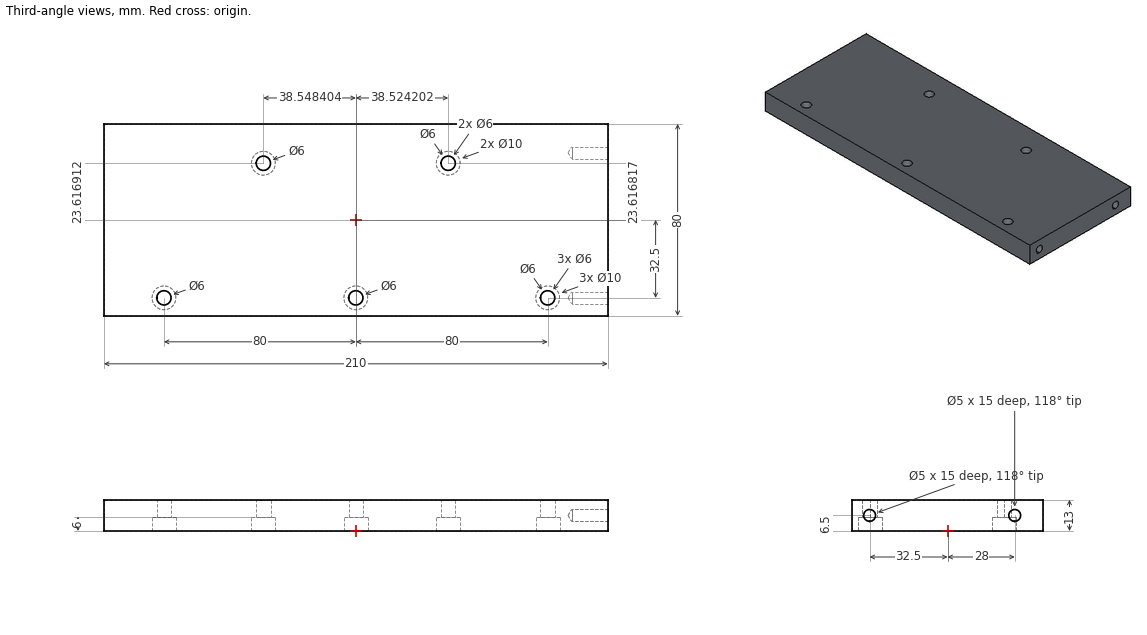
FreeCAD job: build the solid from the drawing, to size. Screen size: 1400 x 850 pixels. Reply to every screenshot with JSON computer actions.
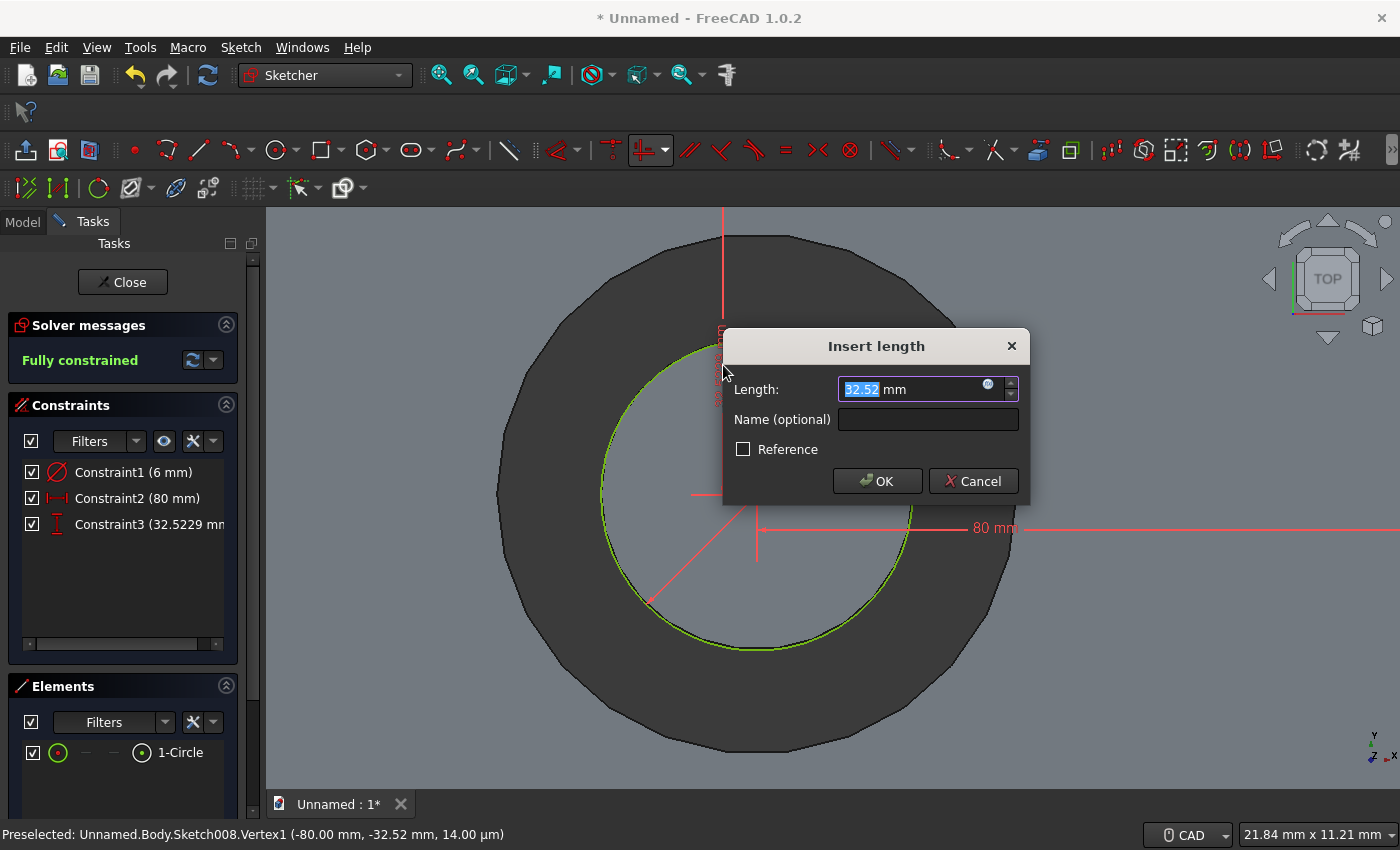
{"action": "type", "text": "32.5"}
{"action": "key", "text": "Return"}
{"action": "key", "text": "Escape"}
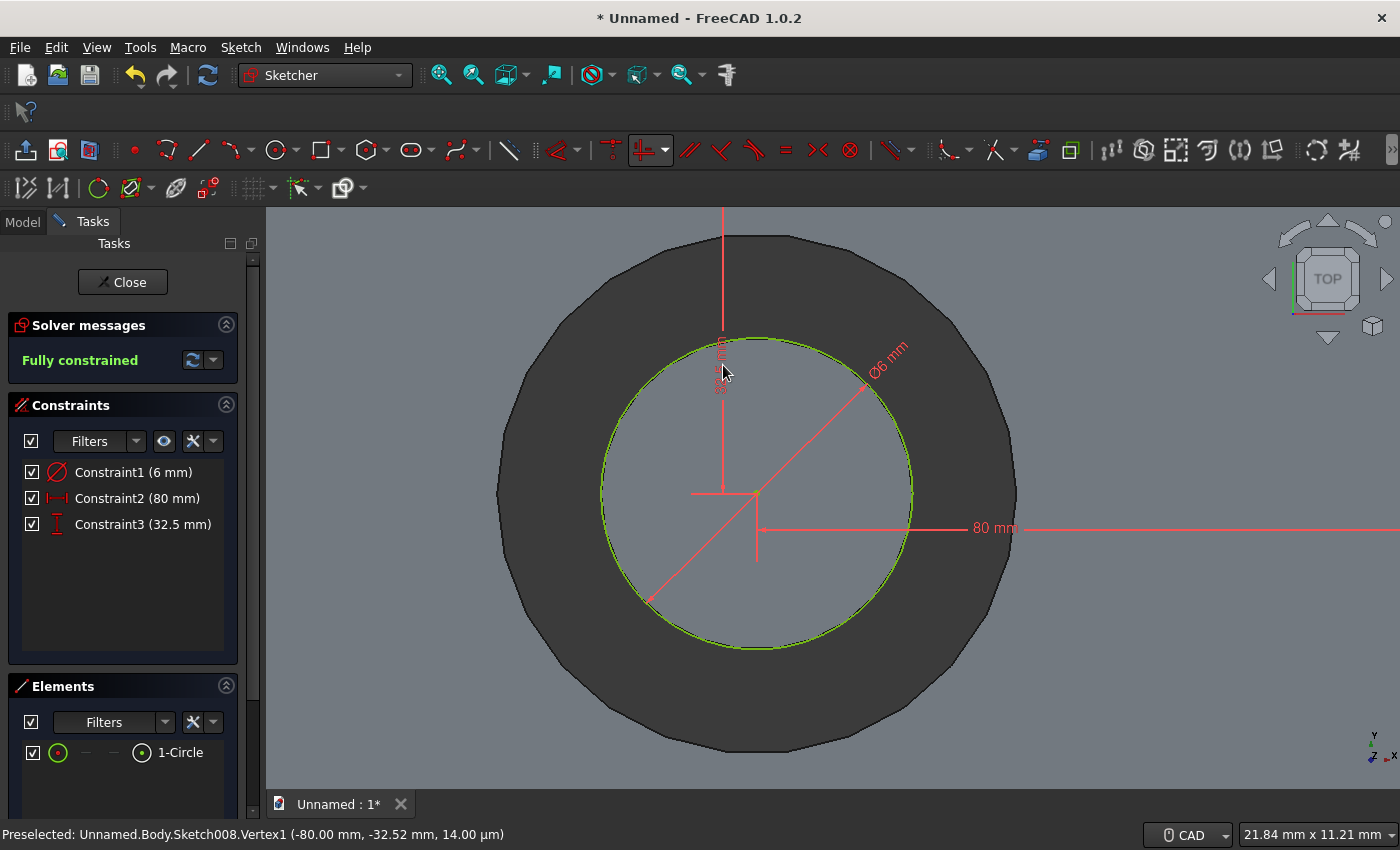
{"action": "left_click", "coordinate": [123, 282]}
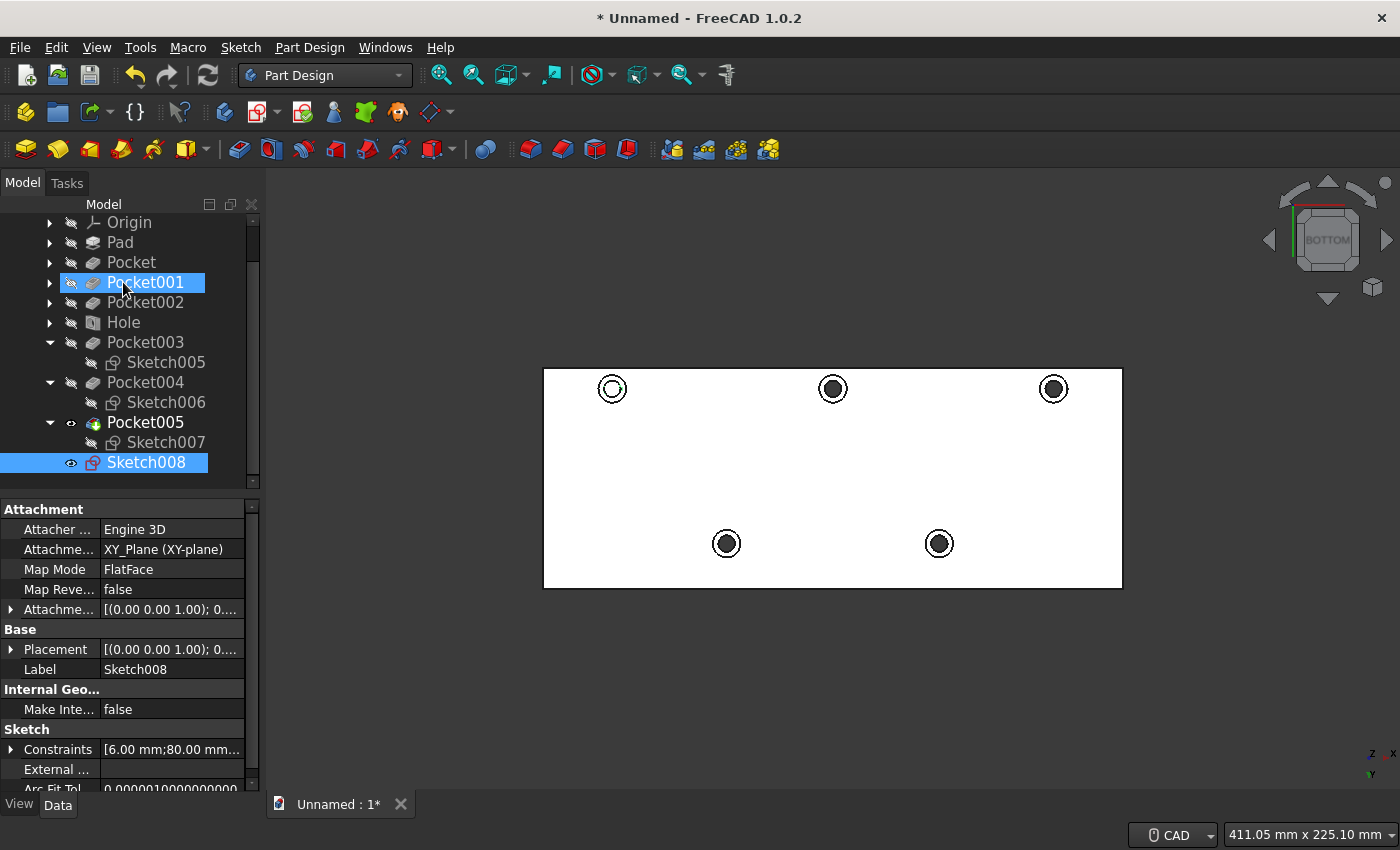
{"action": "left_click", "coordinate": [240, 150]}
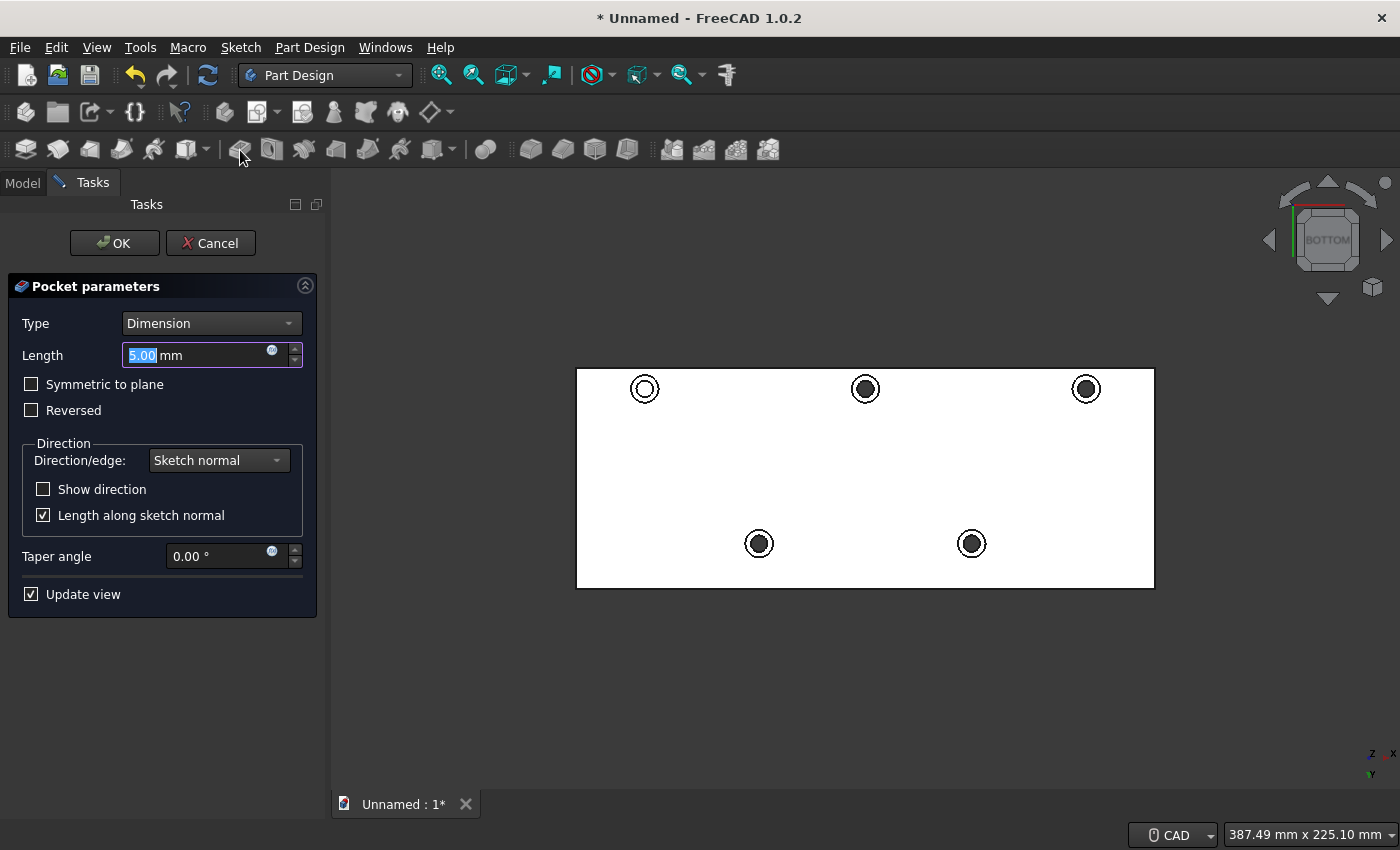
{"action": "left_click", "coordinate": [212, 324]}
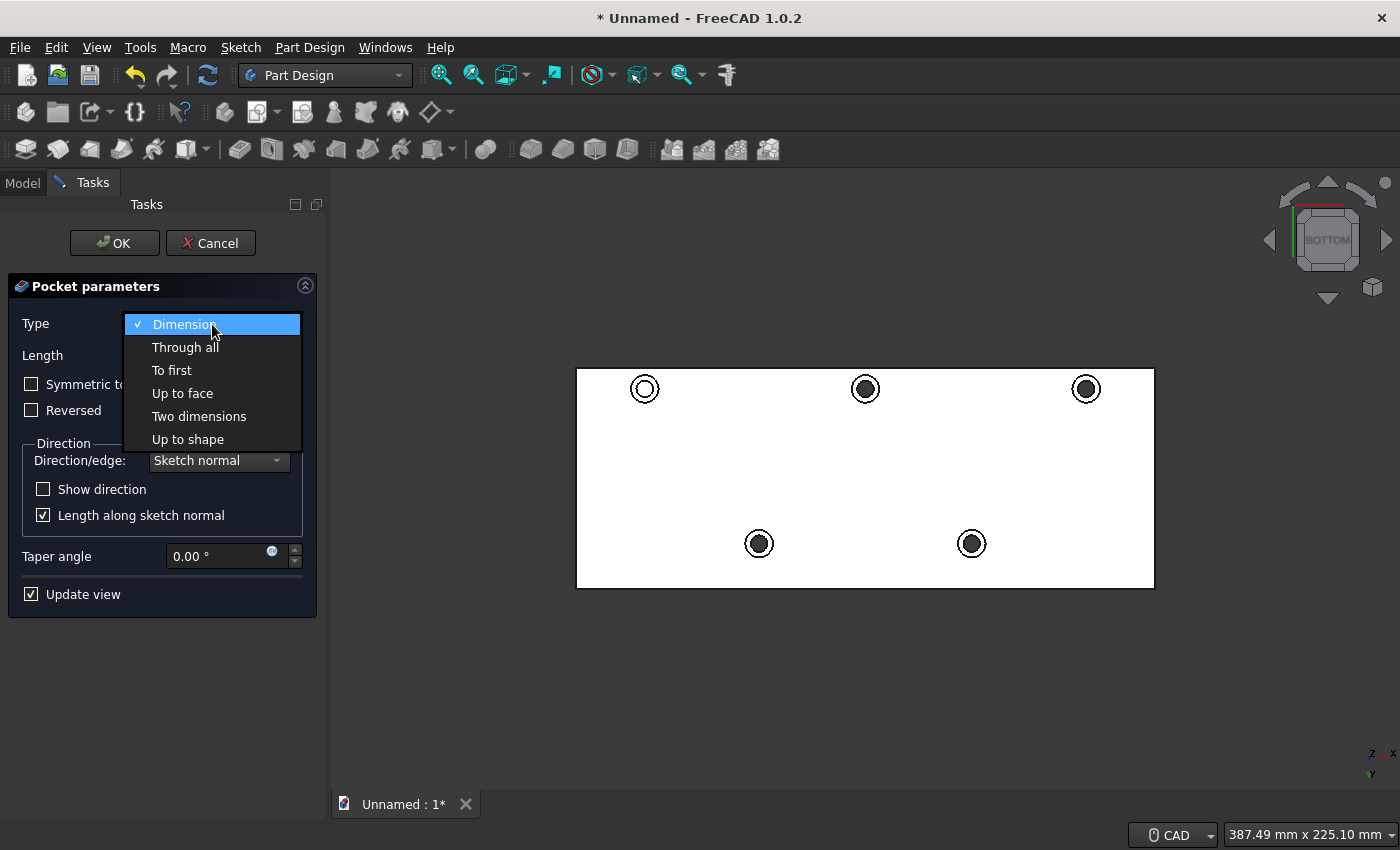
{"action": "left_click", "coordinate": [212, 370]}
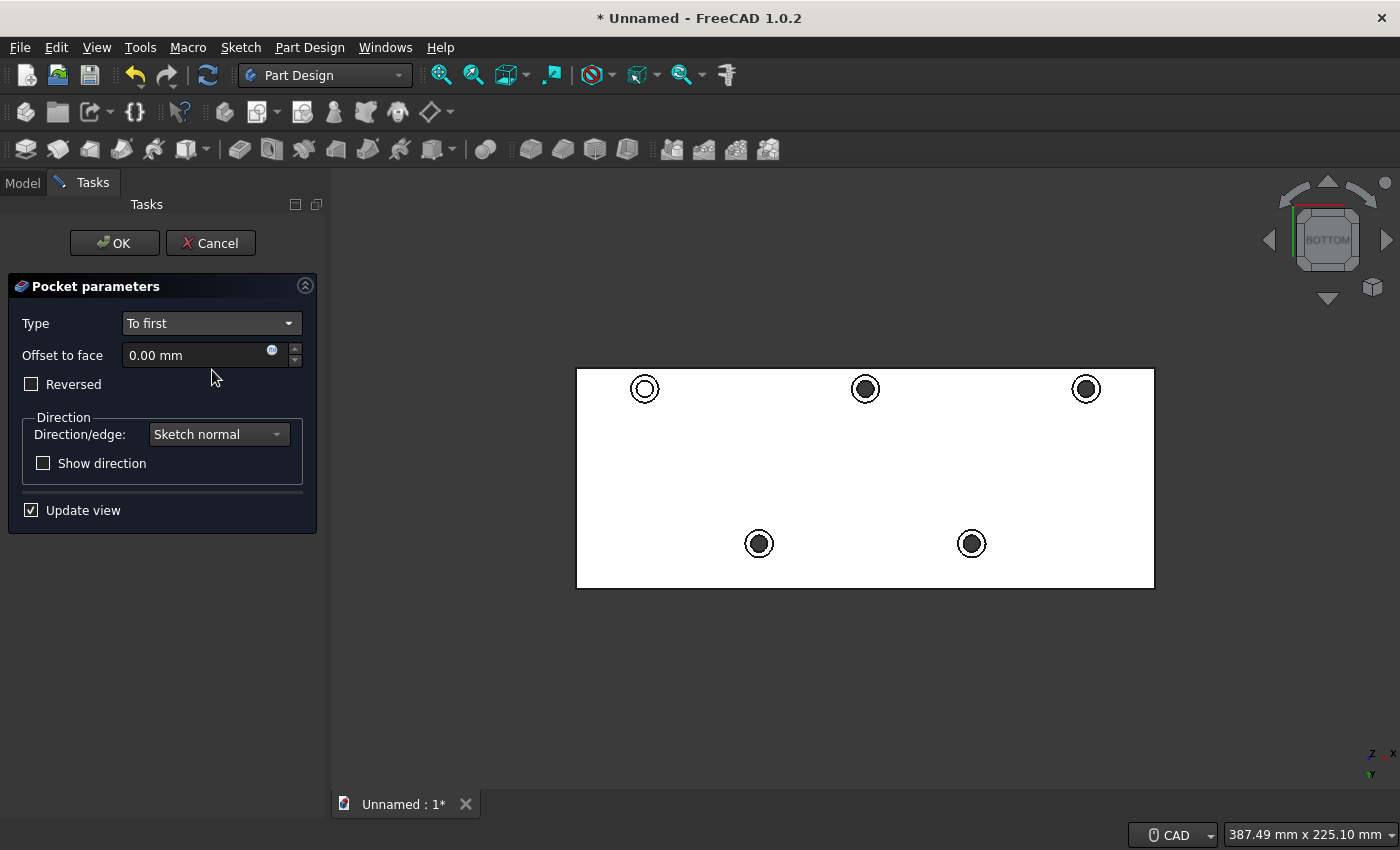
{"action": "left_click", "coordinate": [30, 384]}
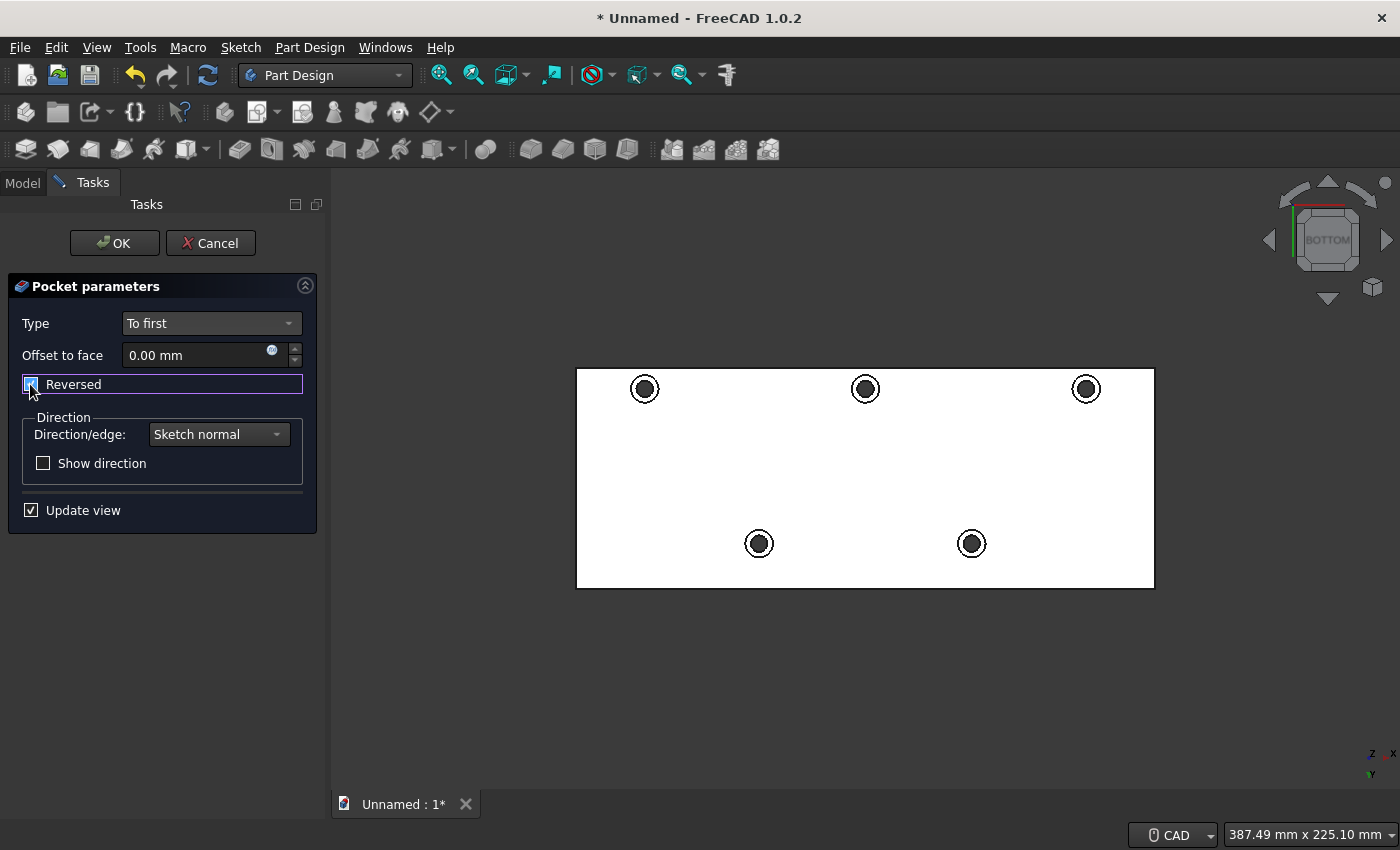
{"action": "left_click", "coordinate": [115, 243]}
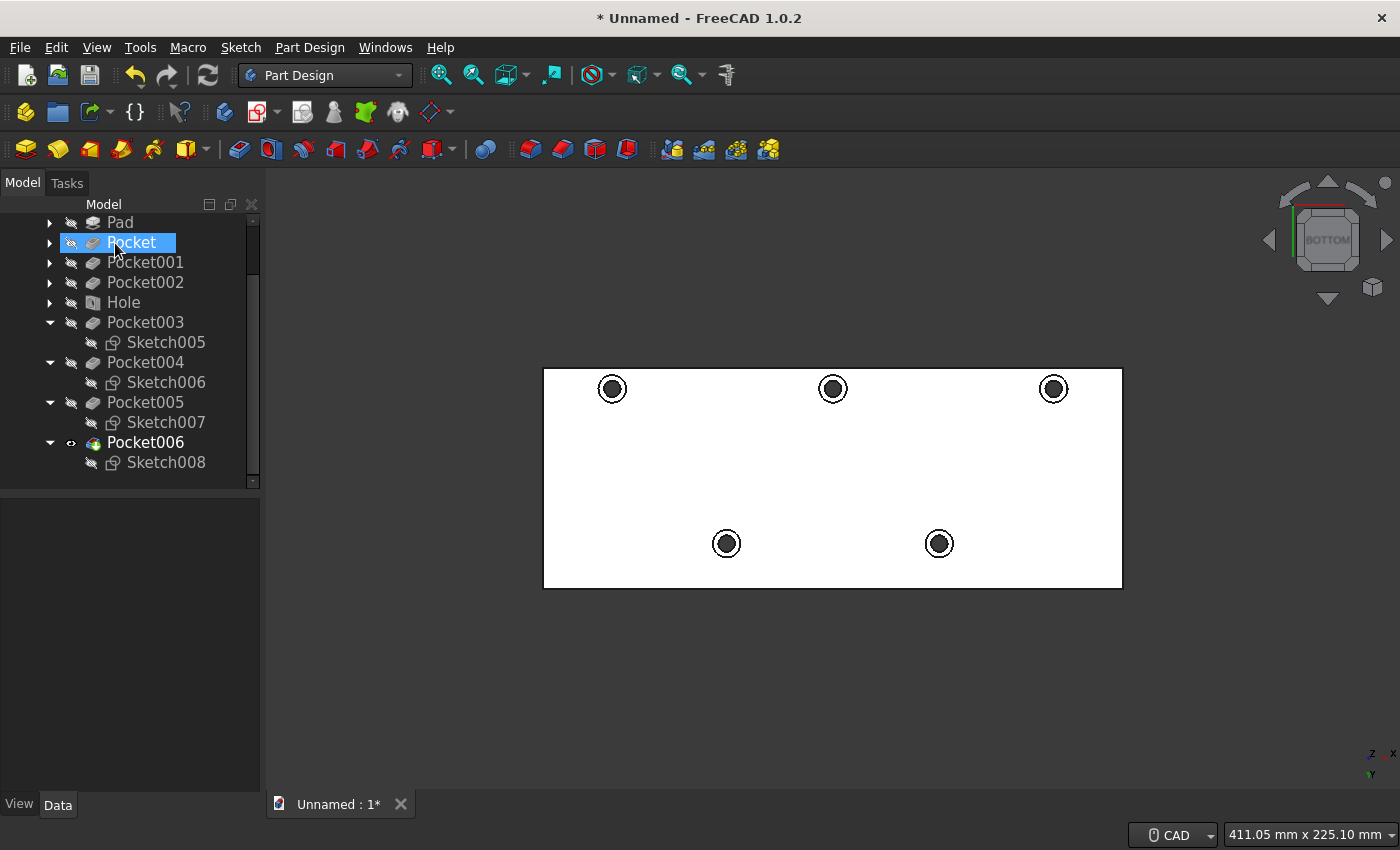
{"action": "key", "text": "0"}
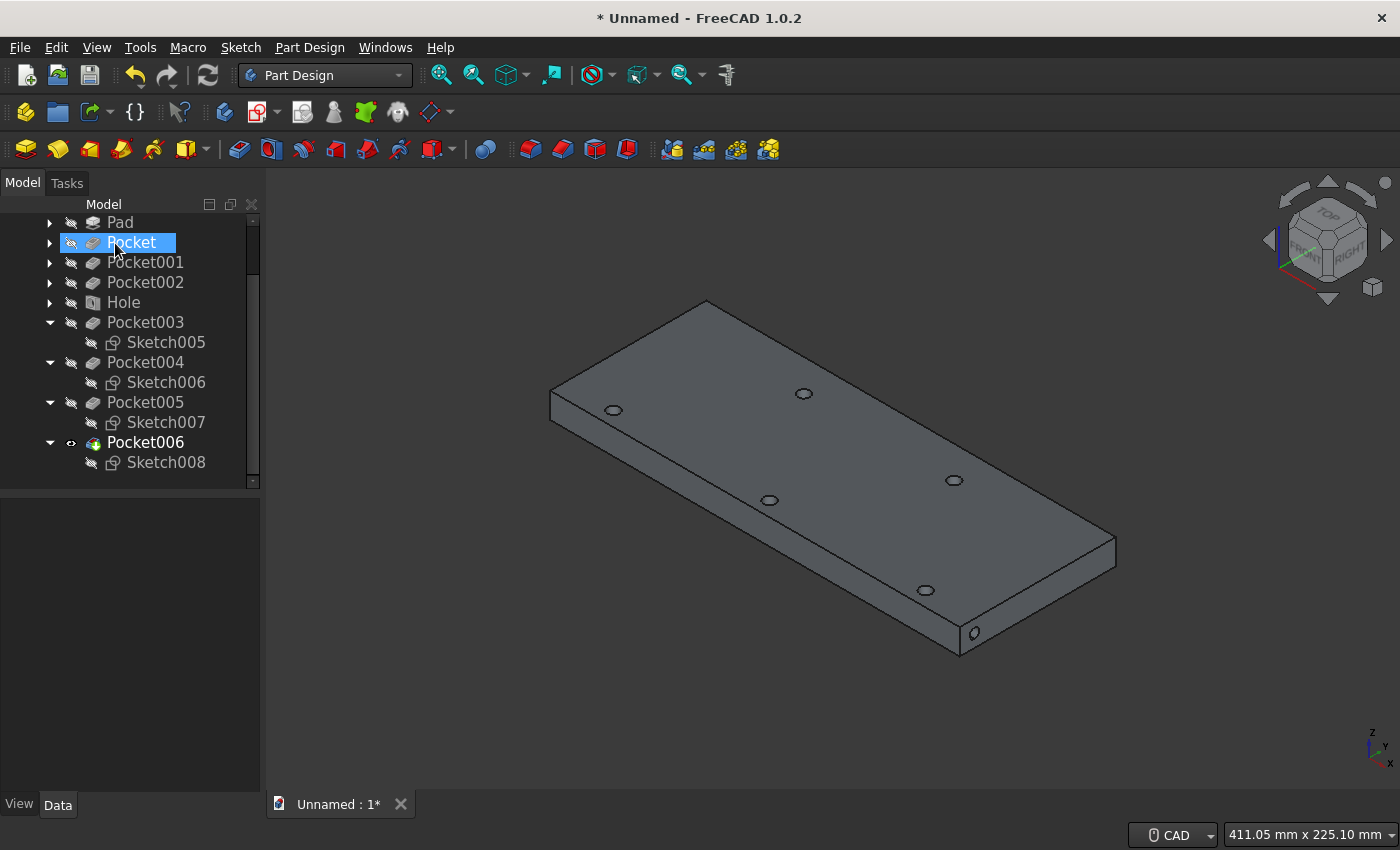
{"action": "left_click", "coordinate": [1082, 570]}